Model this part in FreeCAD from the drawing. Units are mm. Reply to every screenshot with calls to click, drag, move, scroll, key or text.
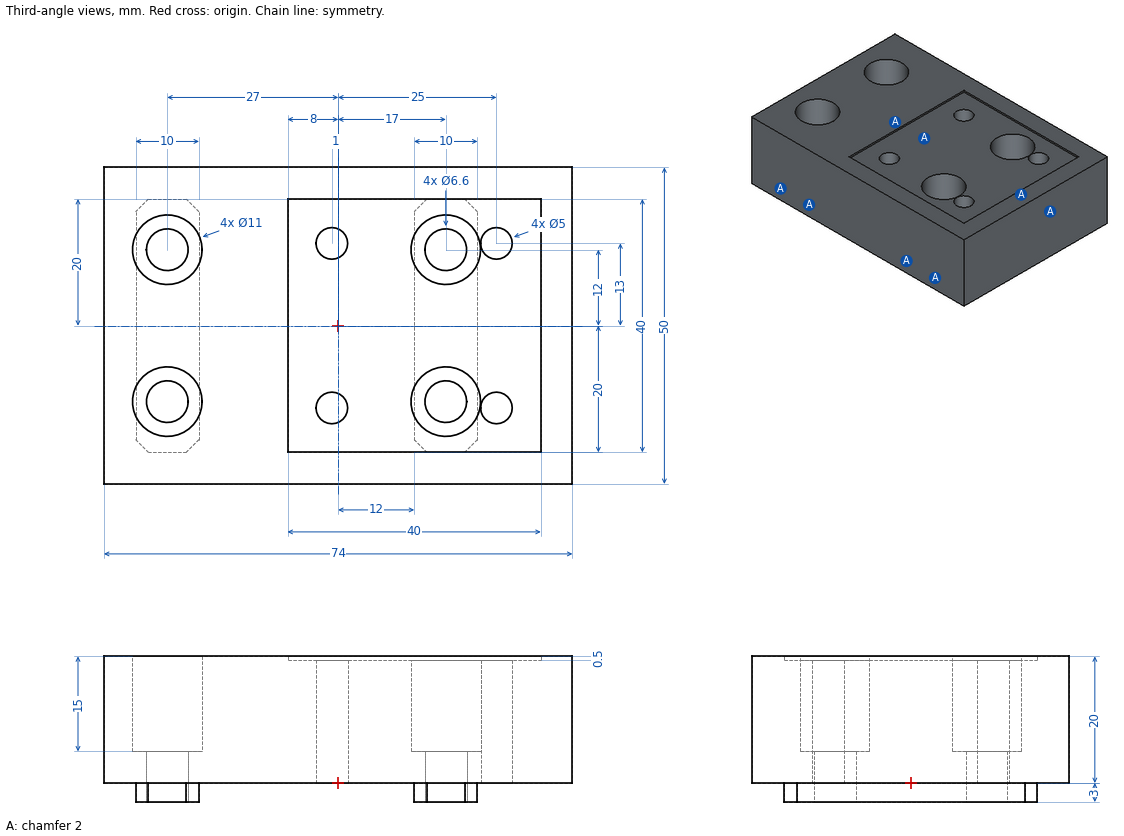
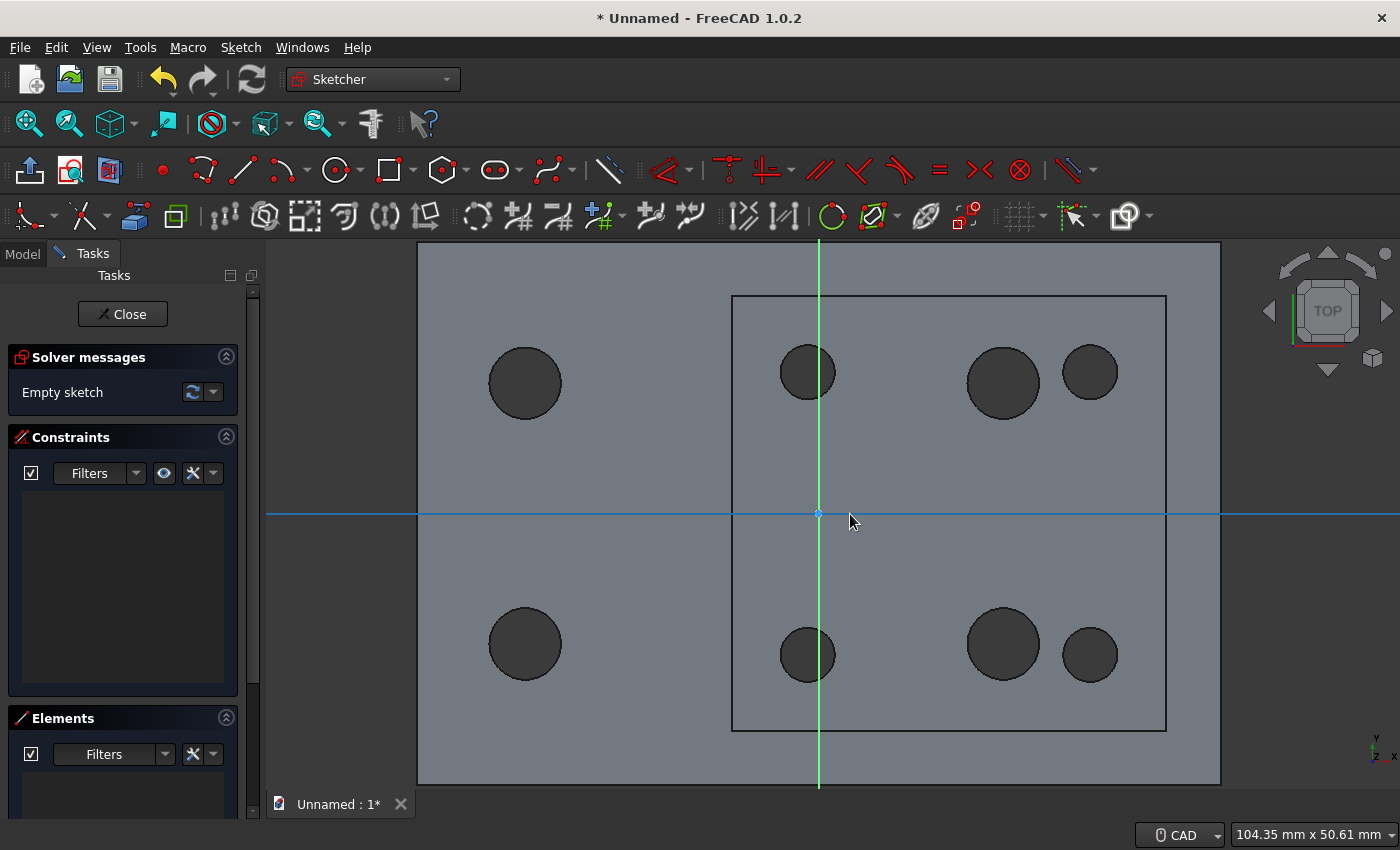
click(336, 170)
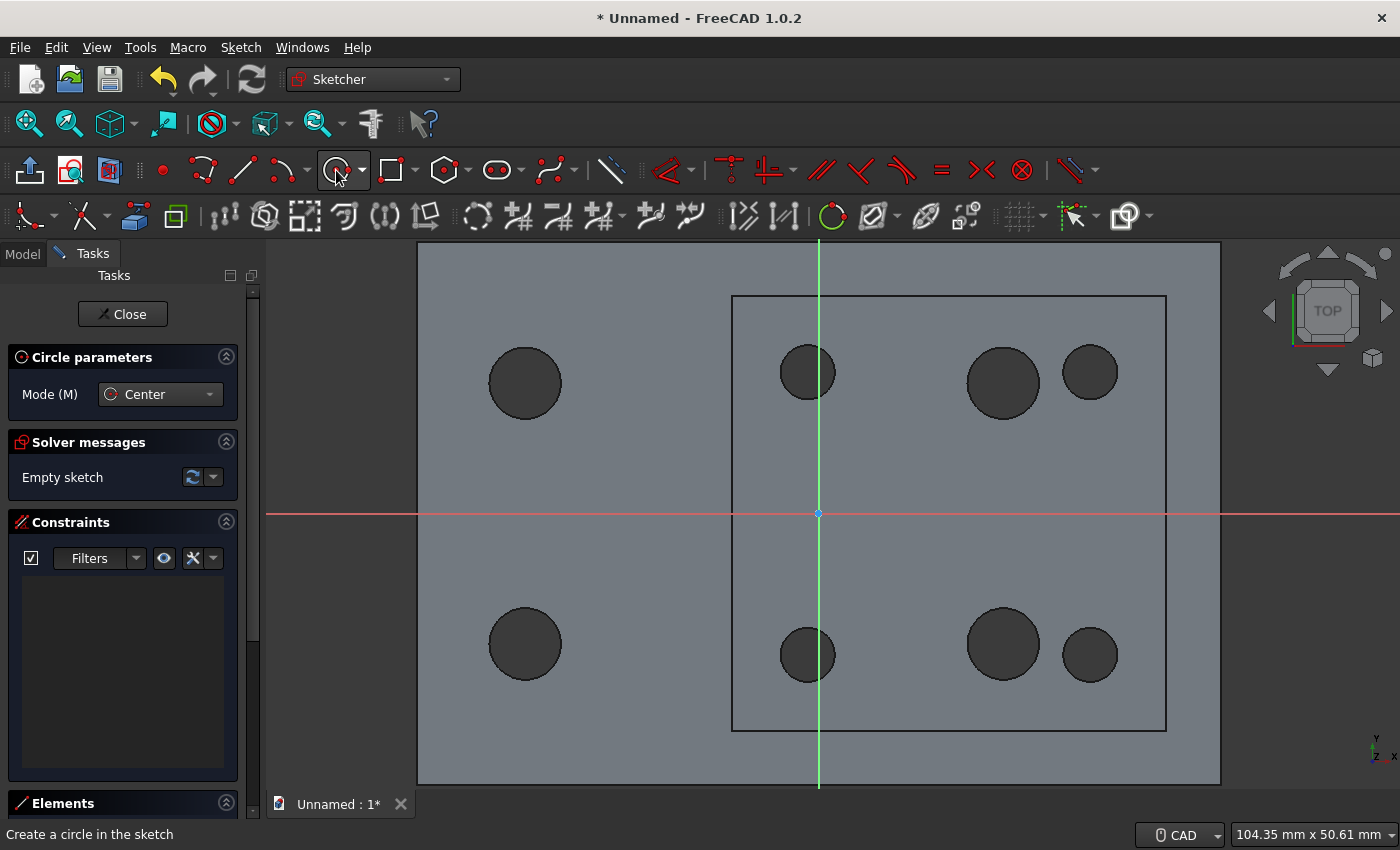
click(525, 383)
move(567, 341)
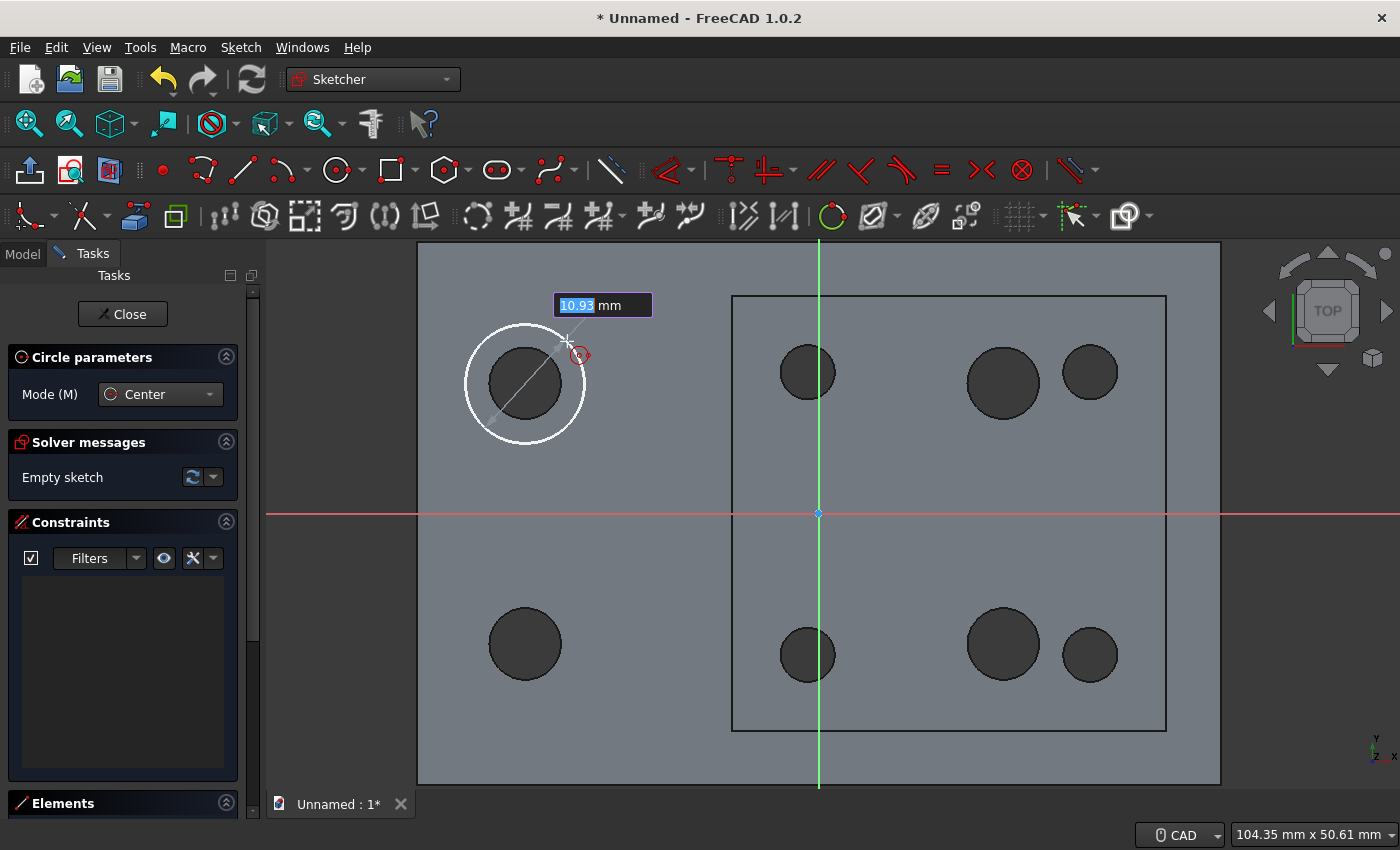
text(11)
key(Return)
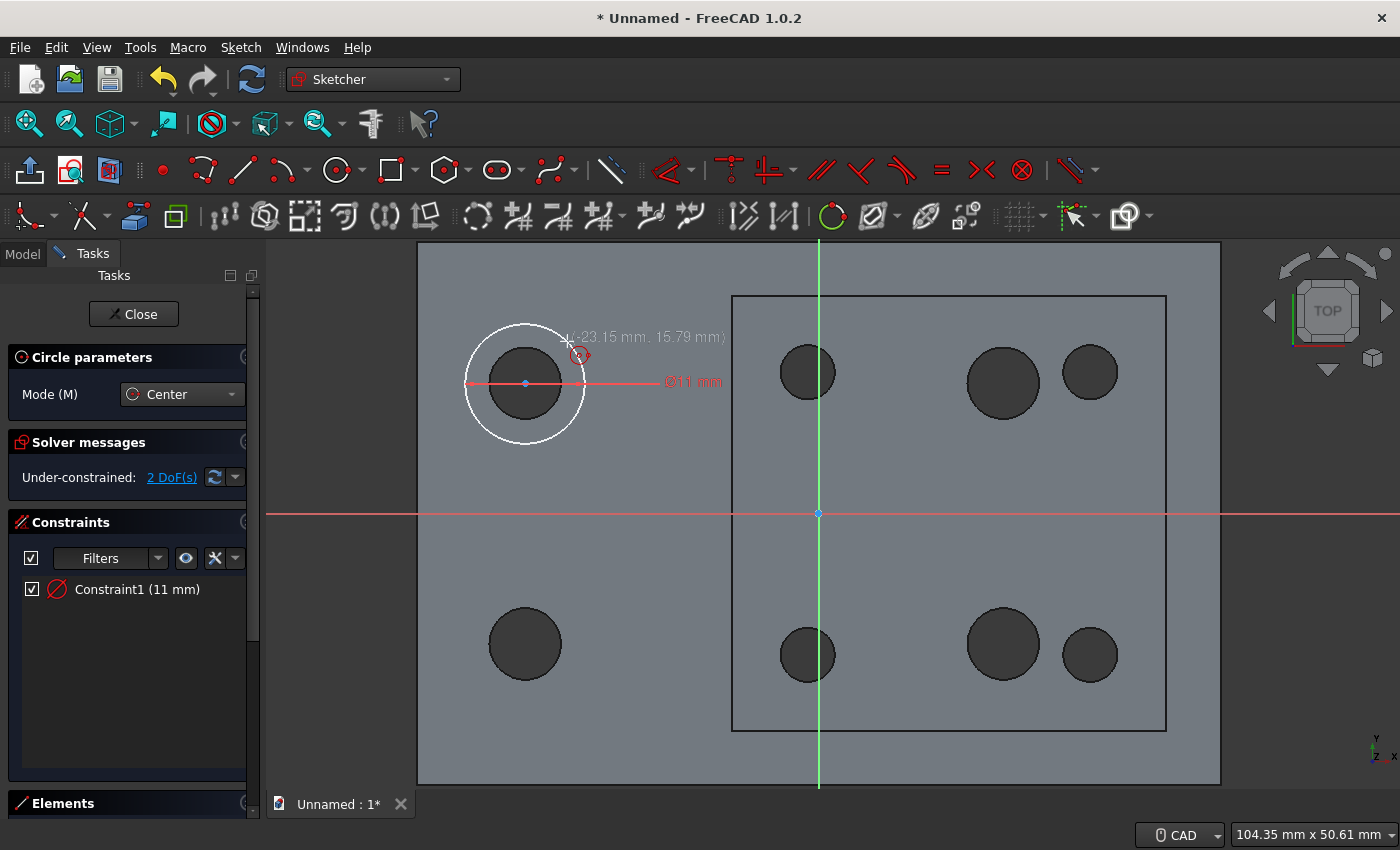
click(525, 644)
move(567, 602)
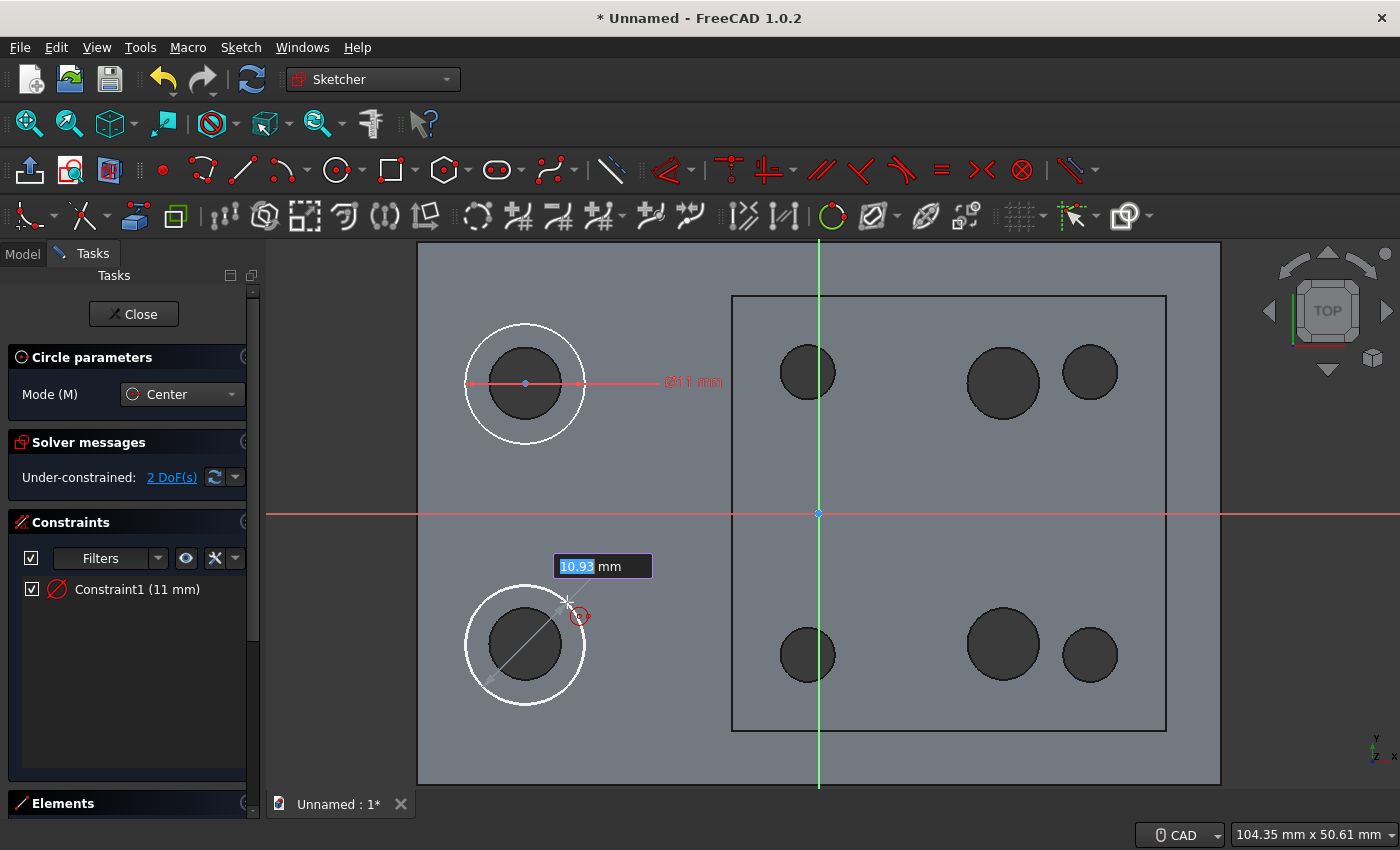
text(11)
key(Return)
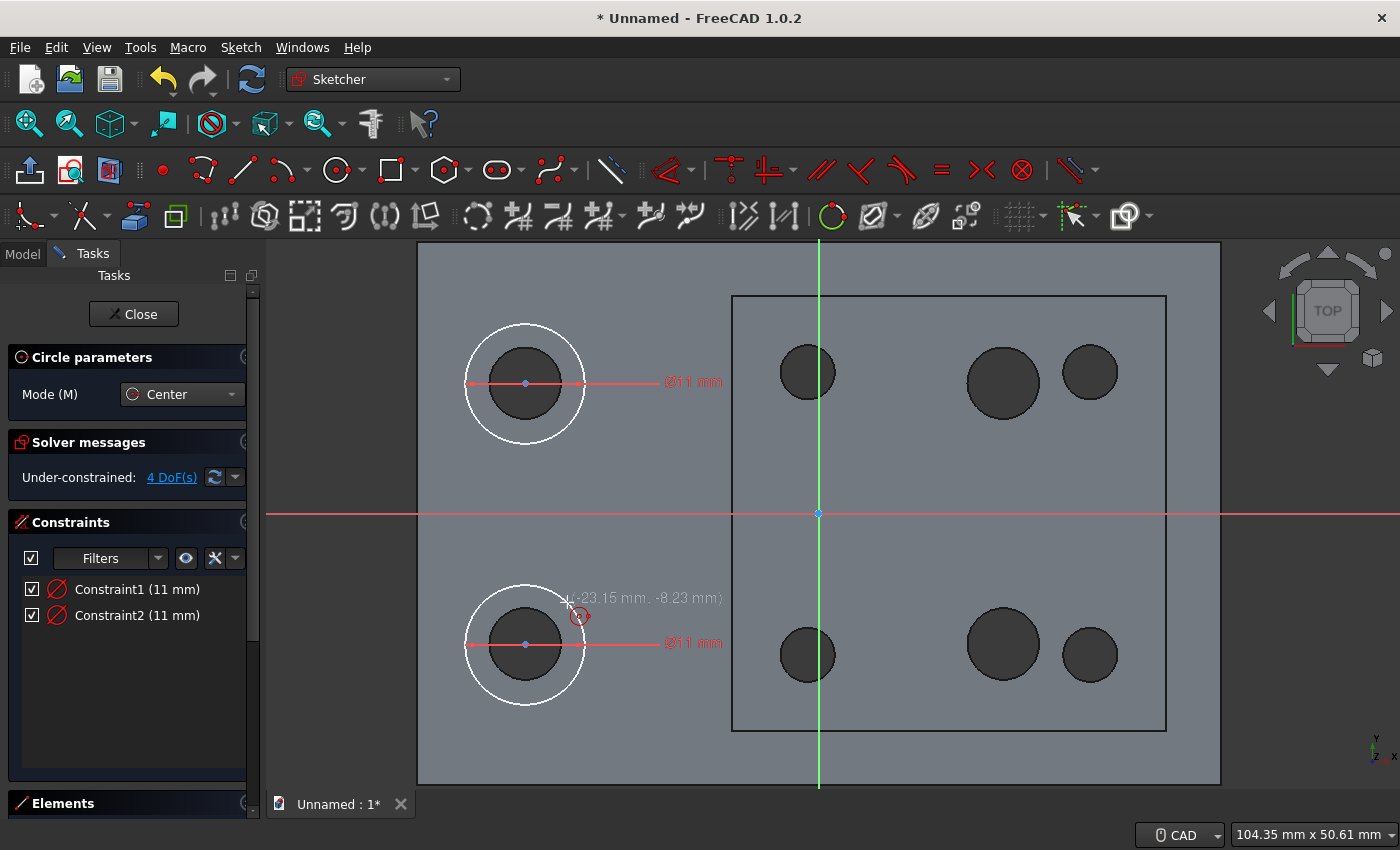
click(1003, 383)
move(1046, 341)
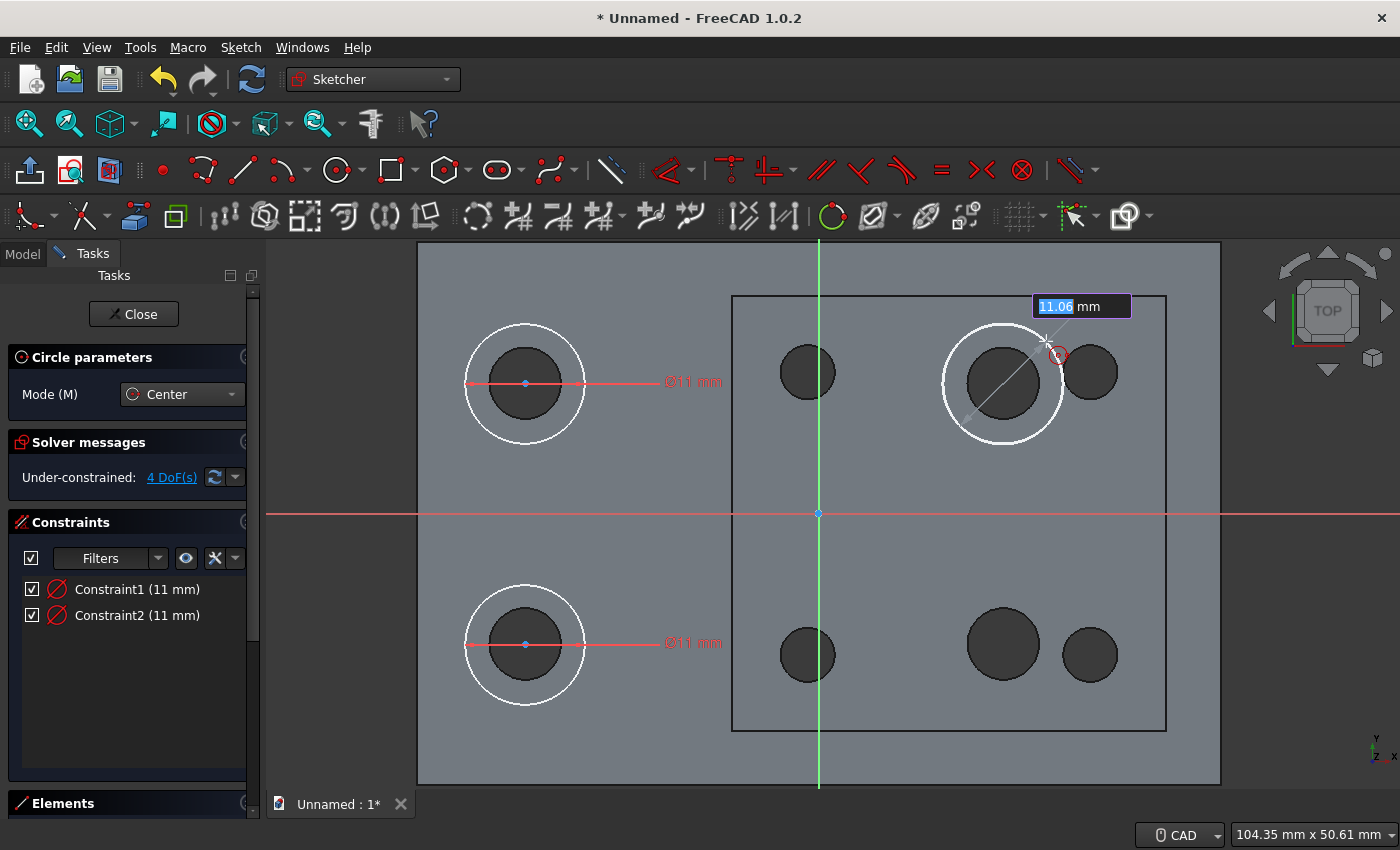
text(11)
key(Return)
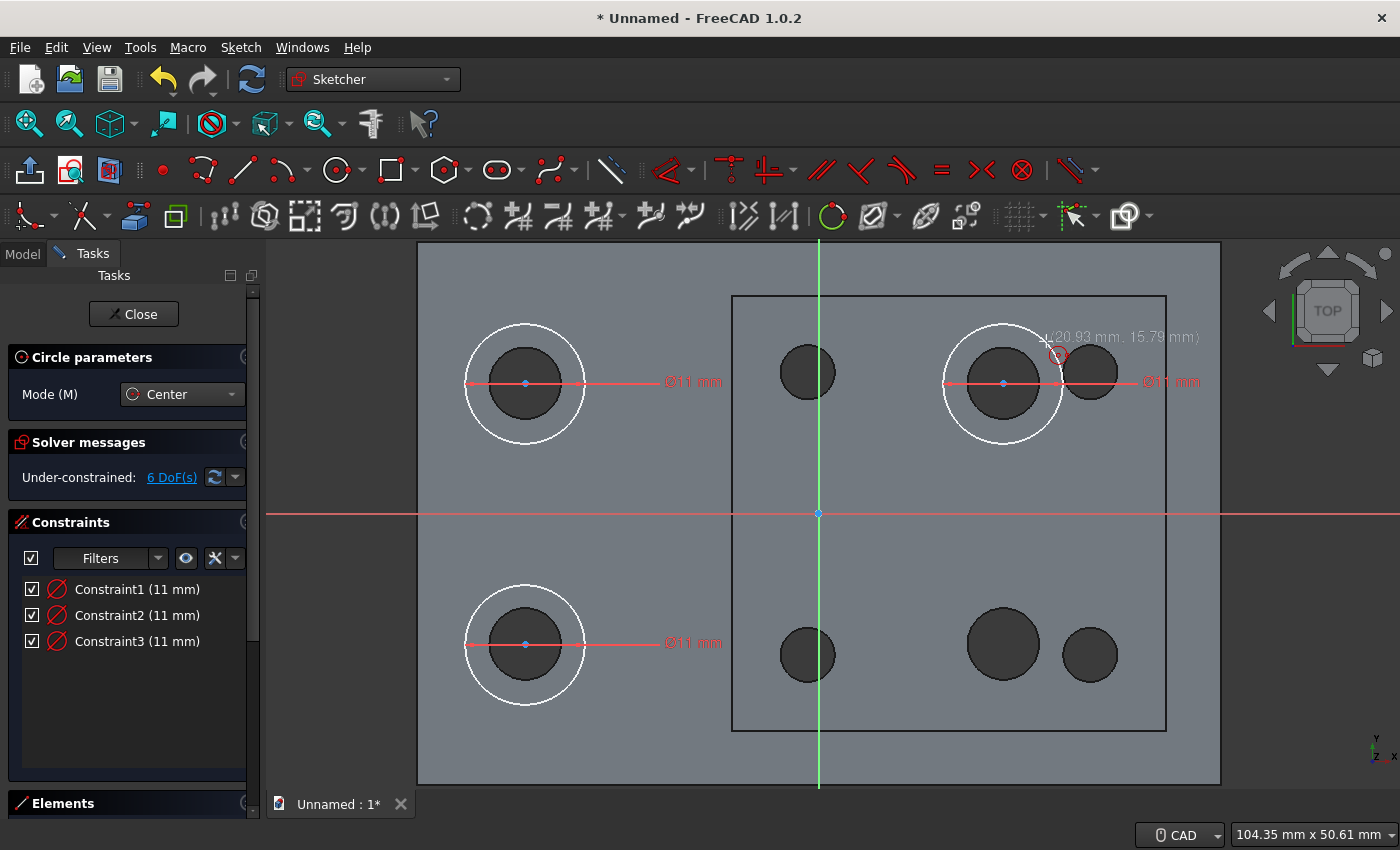
click(1003, 644)
move(1046, 602)